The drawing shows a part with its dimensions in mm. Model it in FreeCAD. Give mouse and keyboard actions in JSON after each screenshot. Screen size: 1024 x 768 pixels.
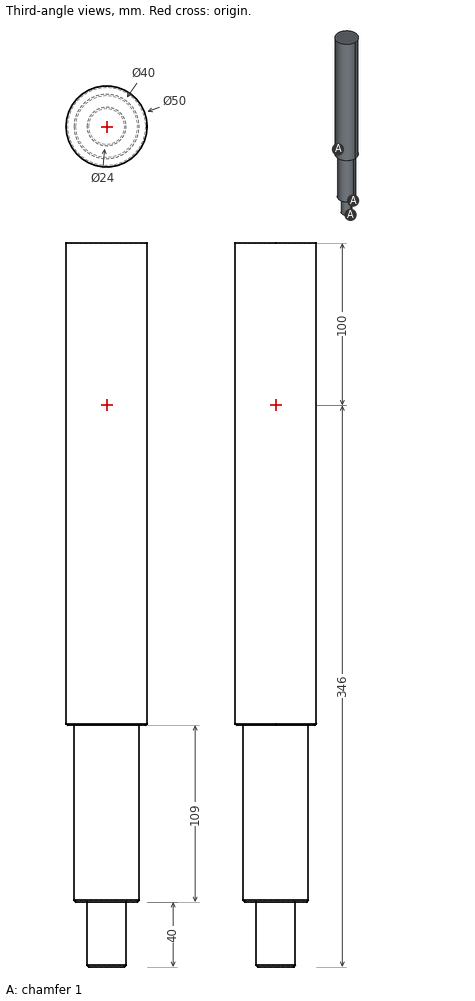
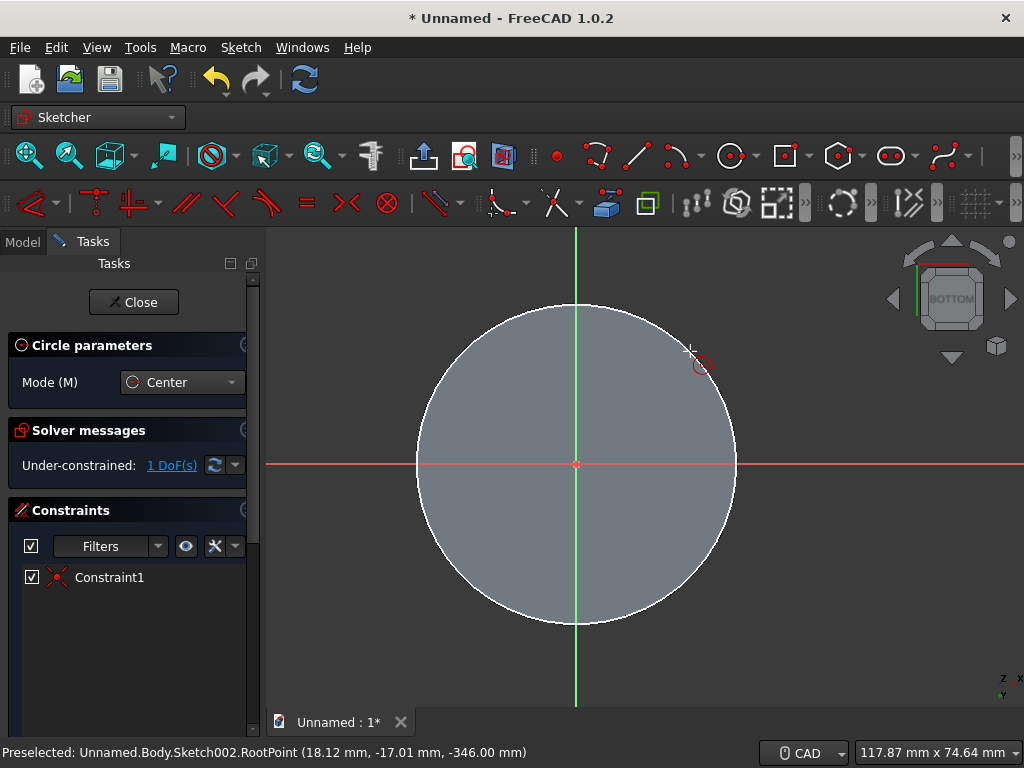
{"action": "left_click", "coordinate": [576, 464]}
{"action": "left_click", "coordinate": [631, 410]}
{"action": "key", "text": "Escape"}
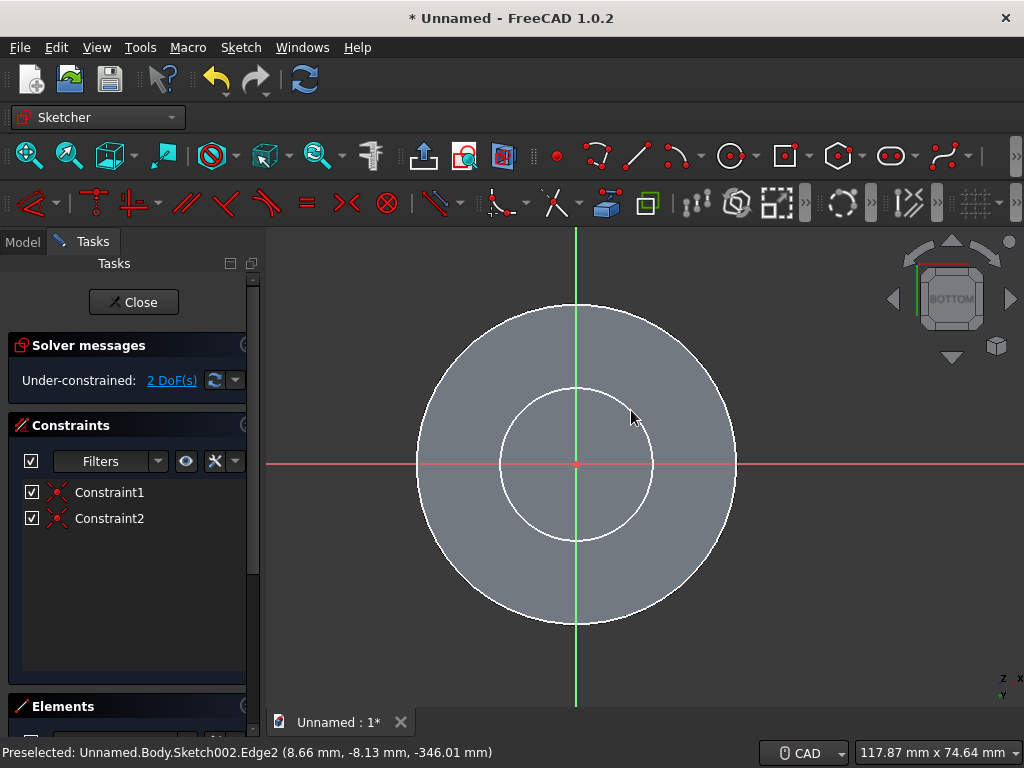
{"action": "left_click", "coordinate": [32, 204]}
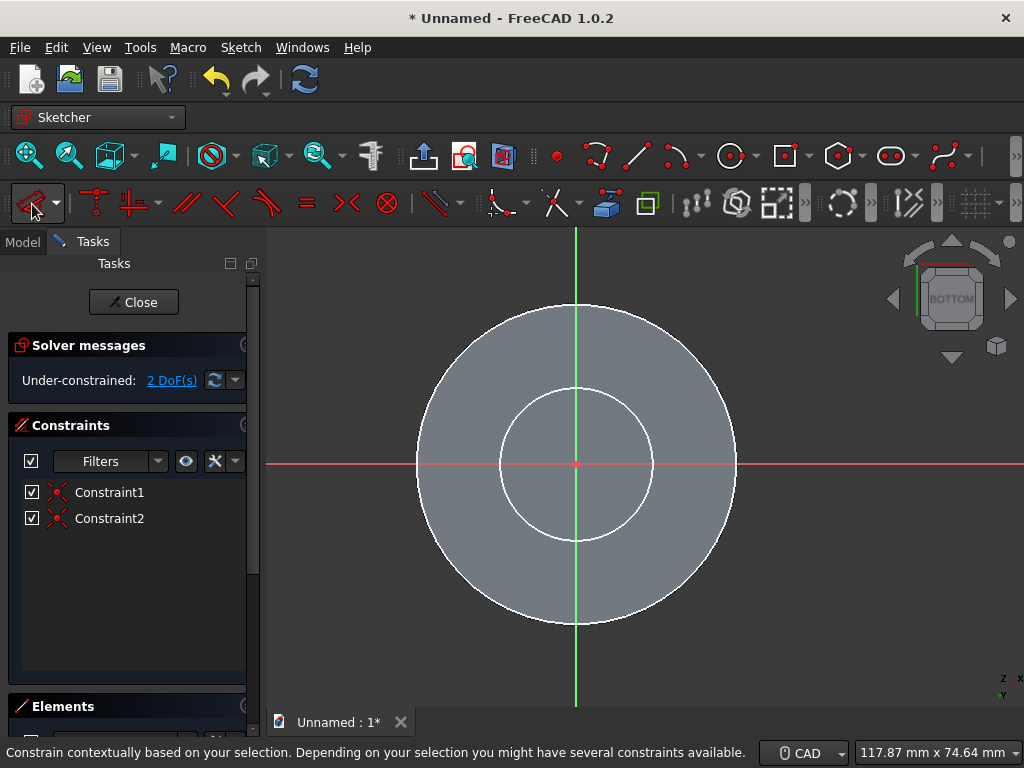
{"action": "left_click", "coordinate": [689, 351]}
{"action": "left_click", "coordinate": [712, 328]}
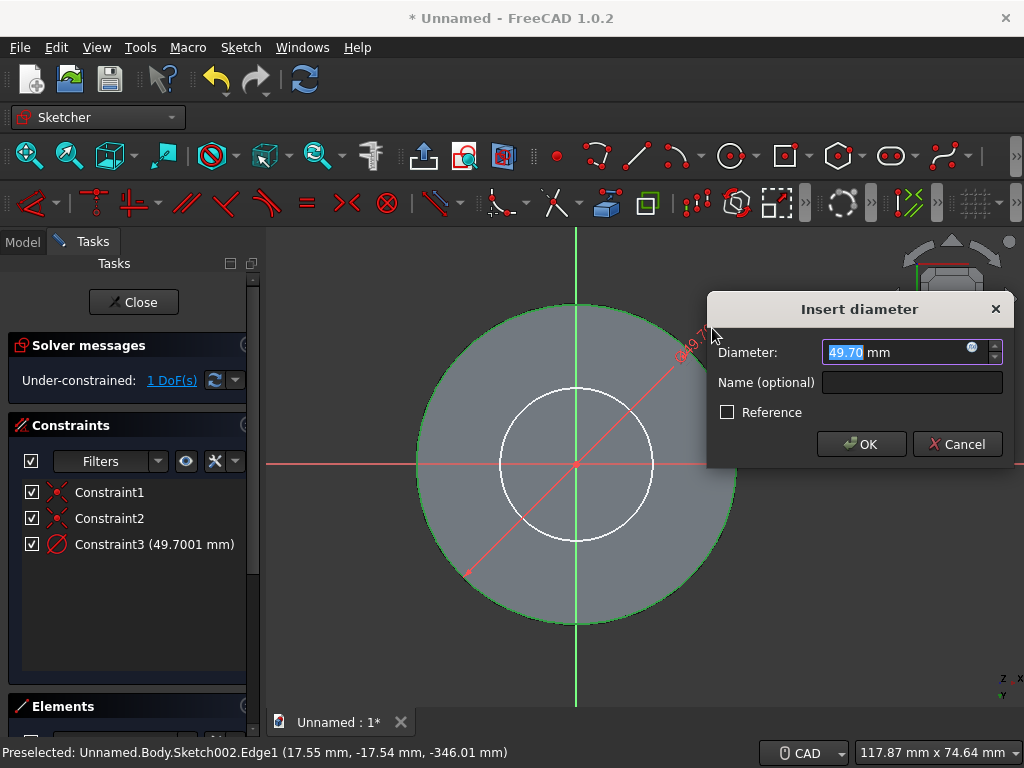
{"action": "type", "text": "50"}
{"action": "key", "text": "Return"}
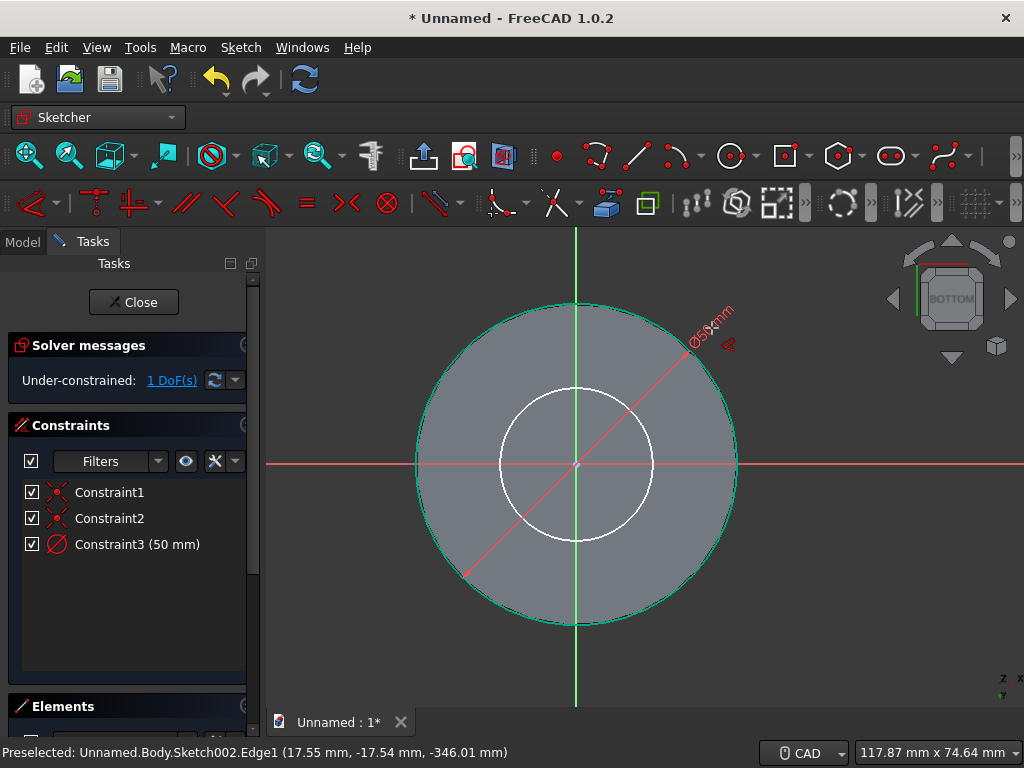
{"action": "left_click", "coordinate": [630, 410]}
{"action": "left_click", "coordinate": [652, 387]}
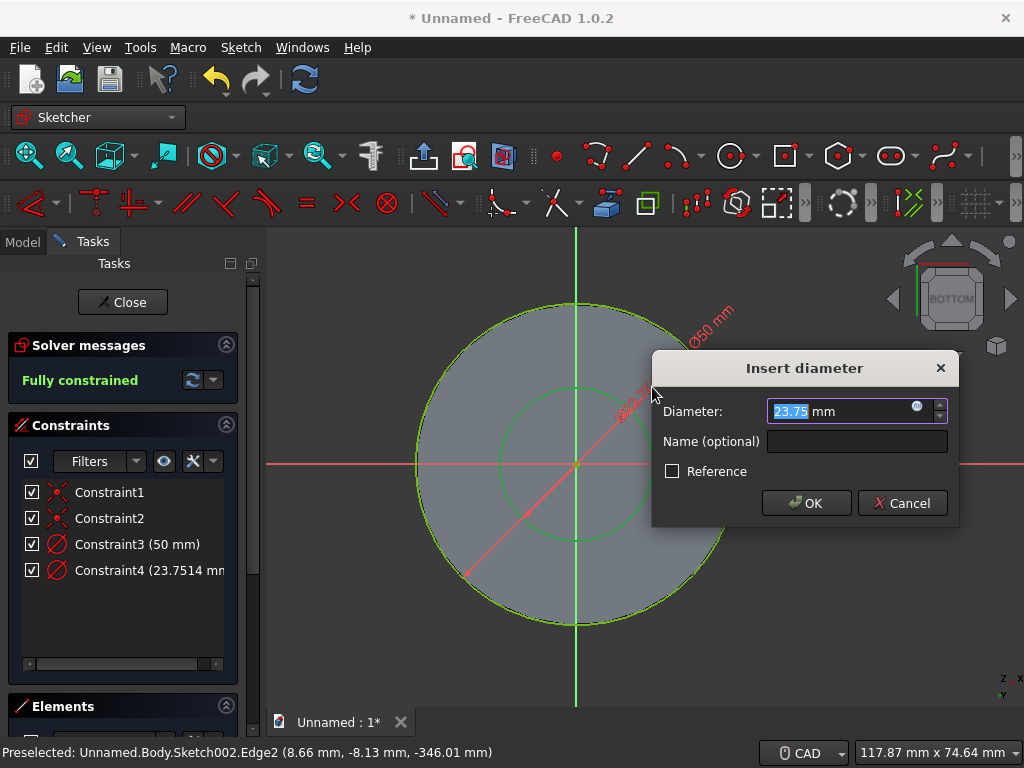
{"action": "type", "text": "24"}
{"action": "key", "text": "Return"}
{"action": "key", "text": "Escape"}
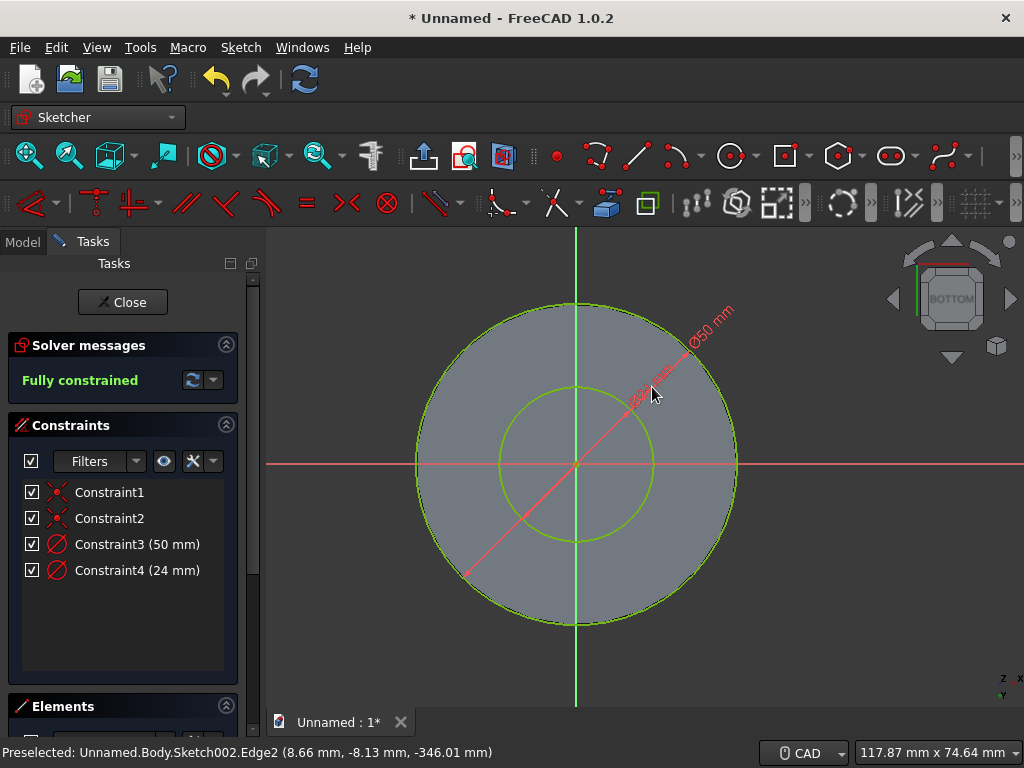
{"action": "left_click", "coordinate": [123, 302]}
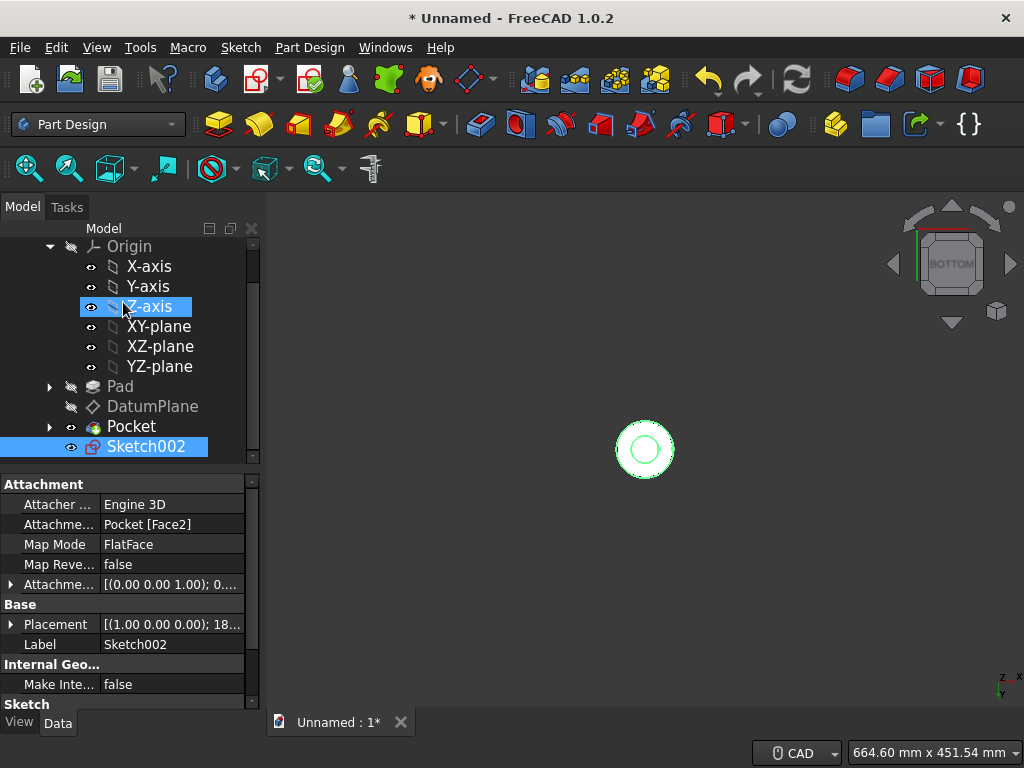
{"action": "left_click", "coordinate": [482, 124]}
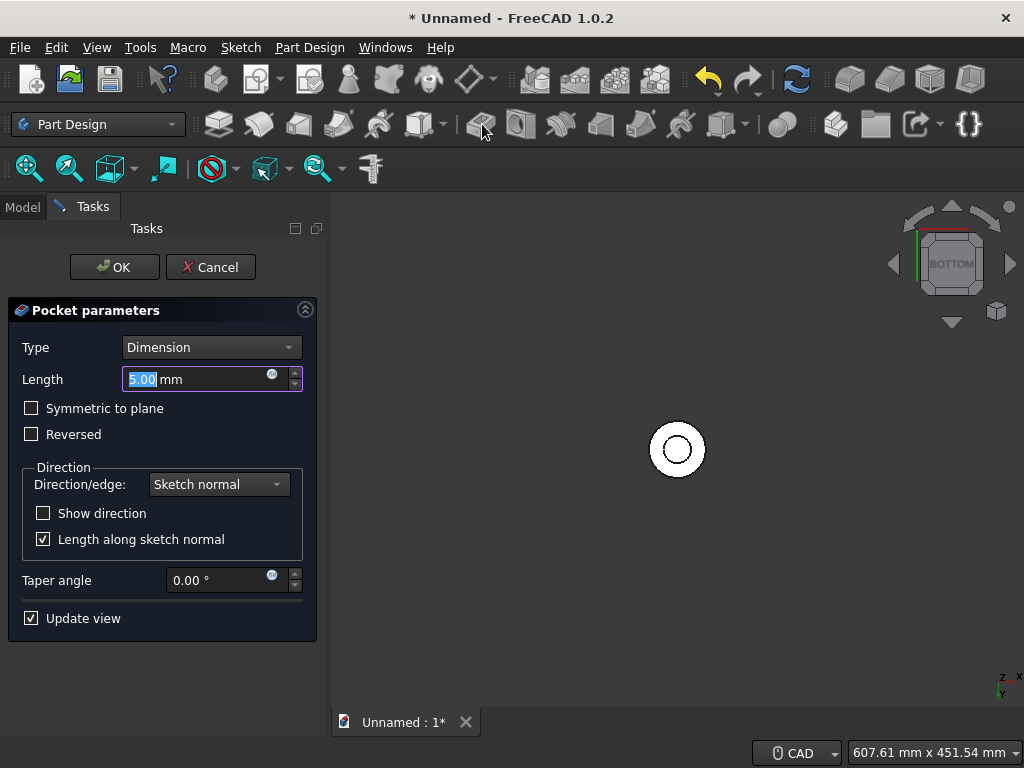
{"action": "type", "text": "40"}
{"action": "key", "text": "Tab"}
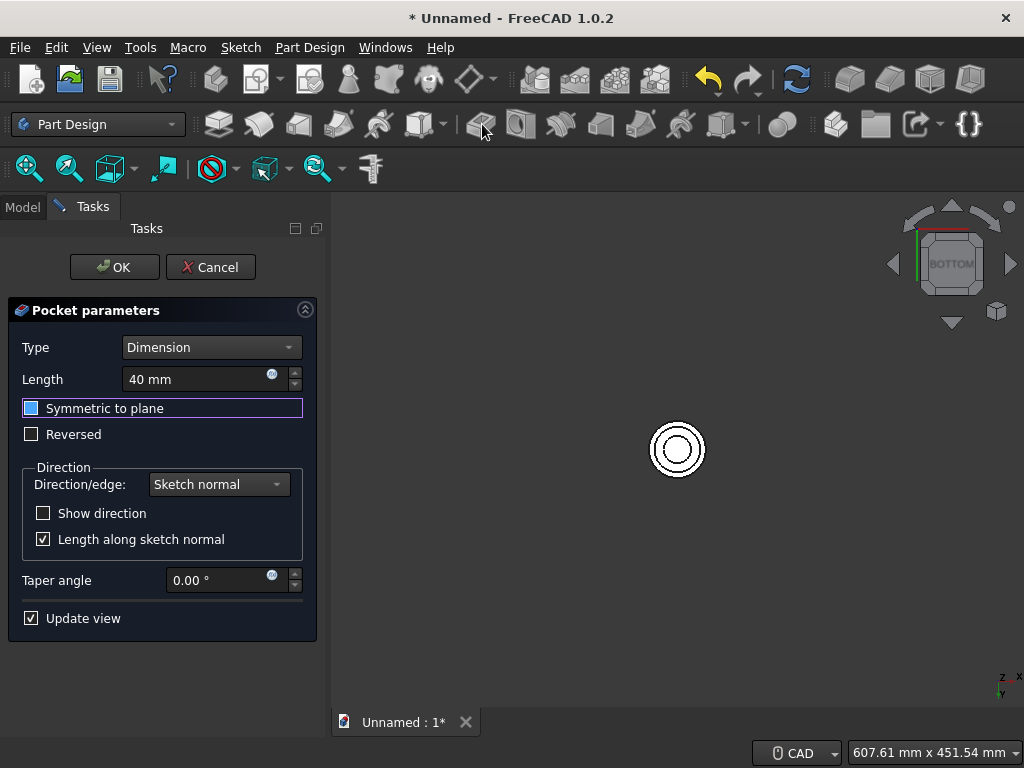
{"action": "left_click", "coordinate": [115, 267]}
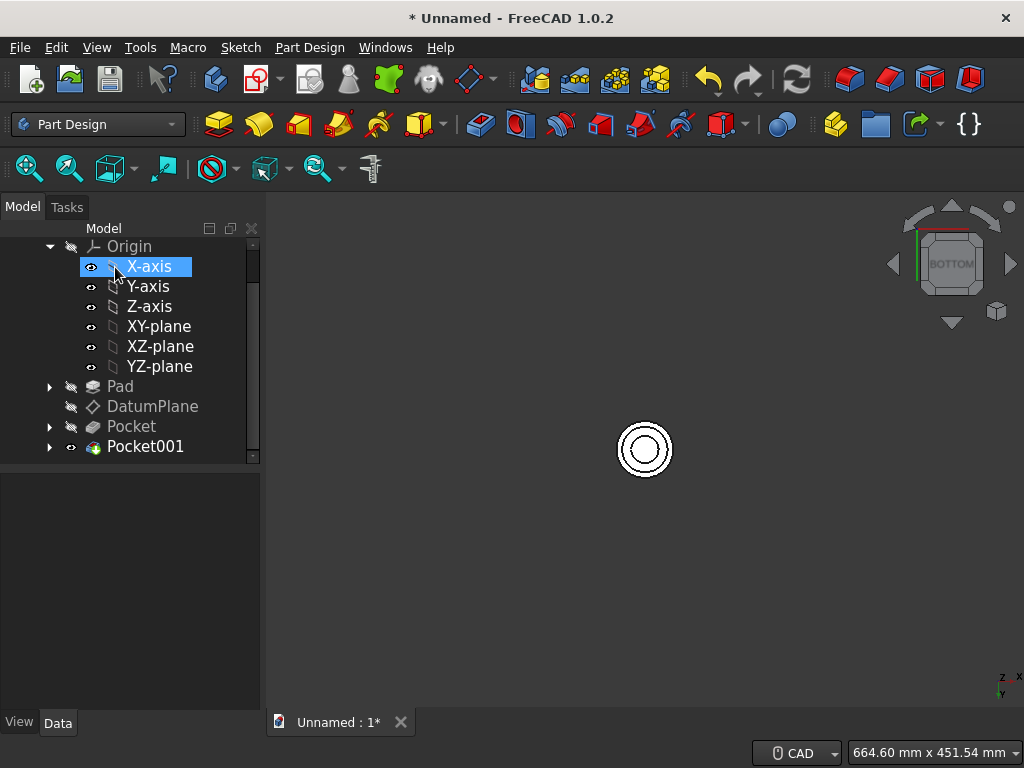
{"action": "left_click", "coordinate": [30, 170]}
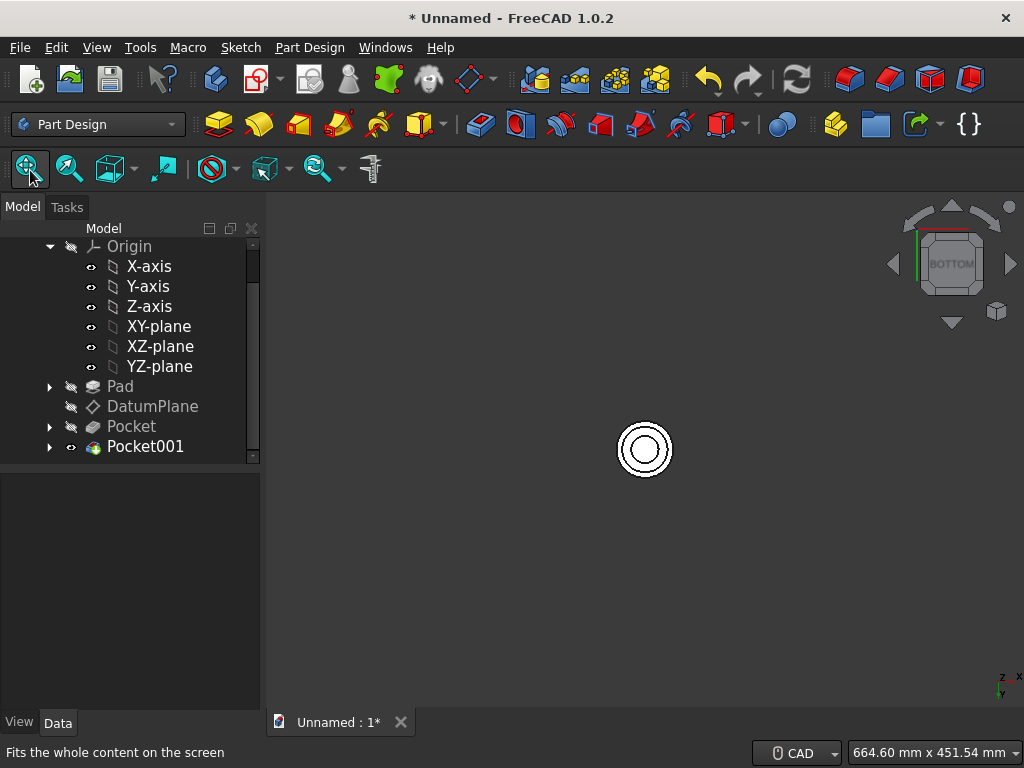
{"action": "left_click", "coordinate": [622, 448]}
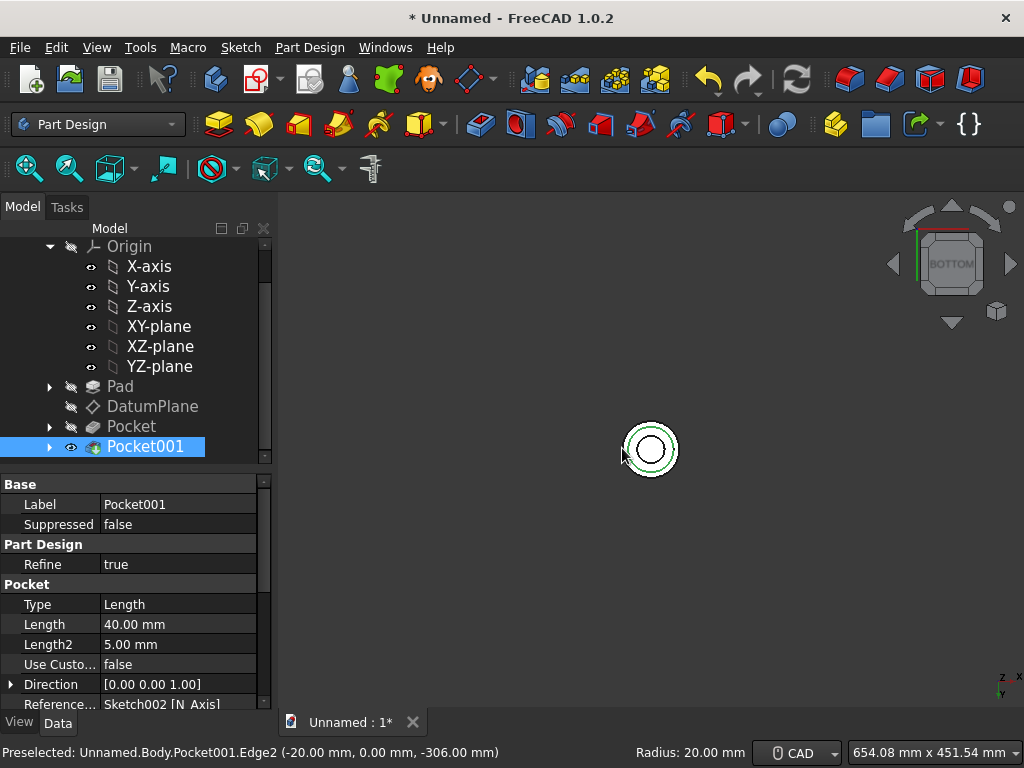
{"action": "left_click", "coordinate": [637, 448], "text": "ctrl"}